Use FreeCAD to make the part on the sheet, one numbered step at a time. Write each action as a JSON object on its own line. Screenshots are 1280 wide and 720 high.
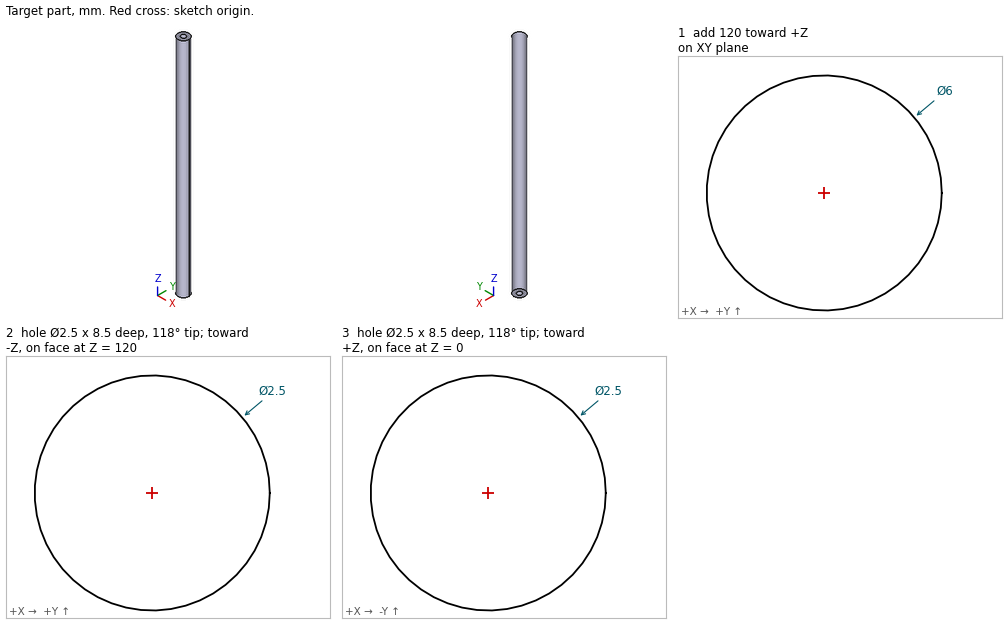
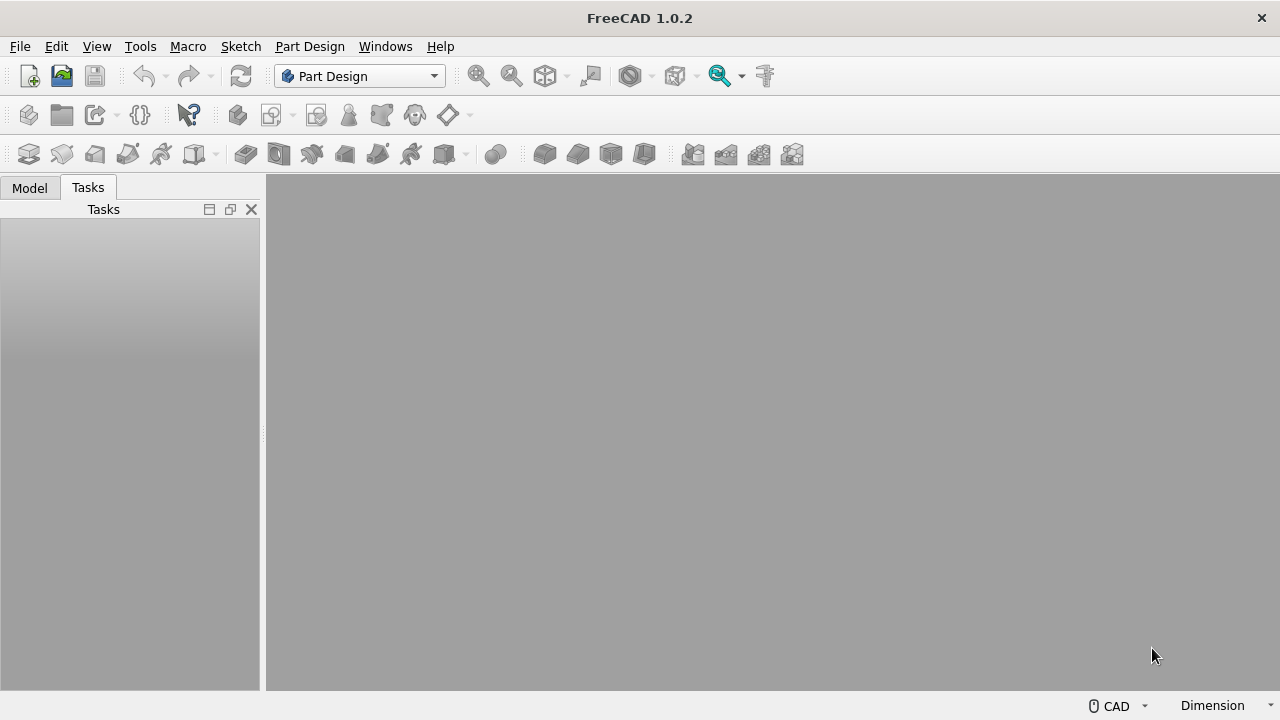
{"action": "left_click", "coordinate": [29, 76]}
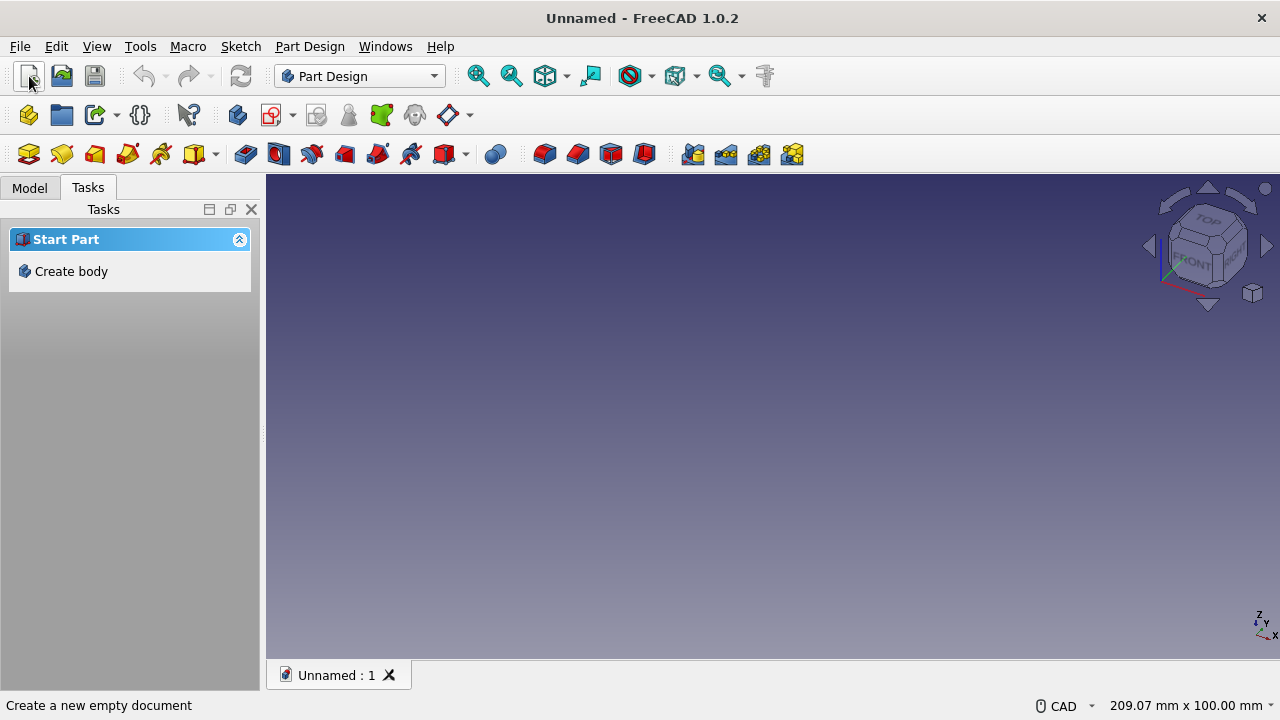
{"action": "left_click", "coordinate": [270, 116]}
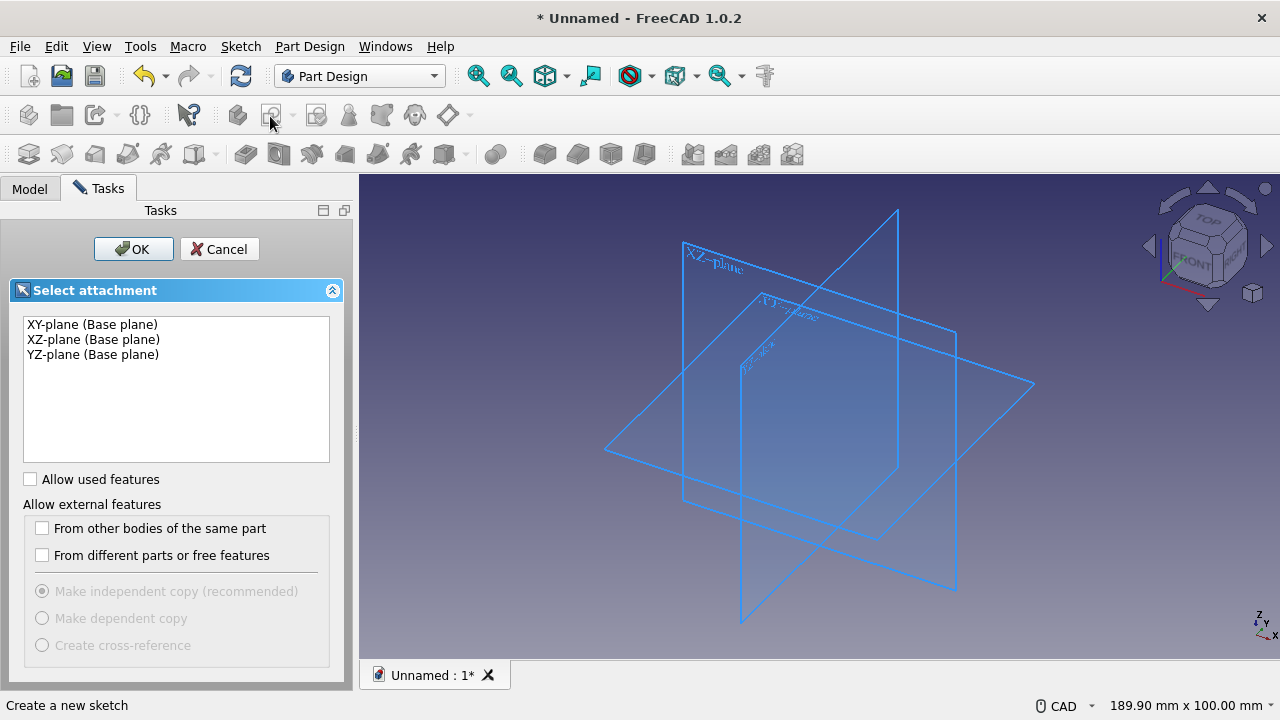
{"action": "left_click", "coordinate": [84, 324]}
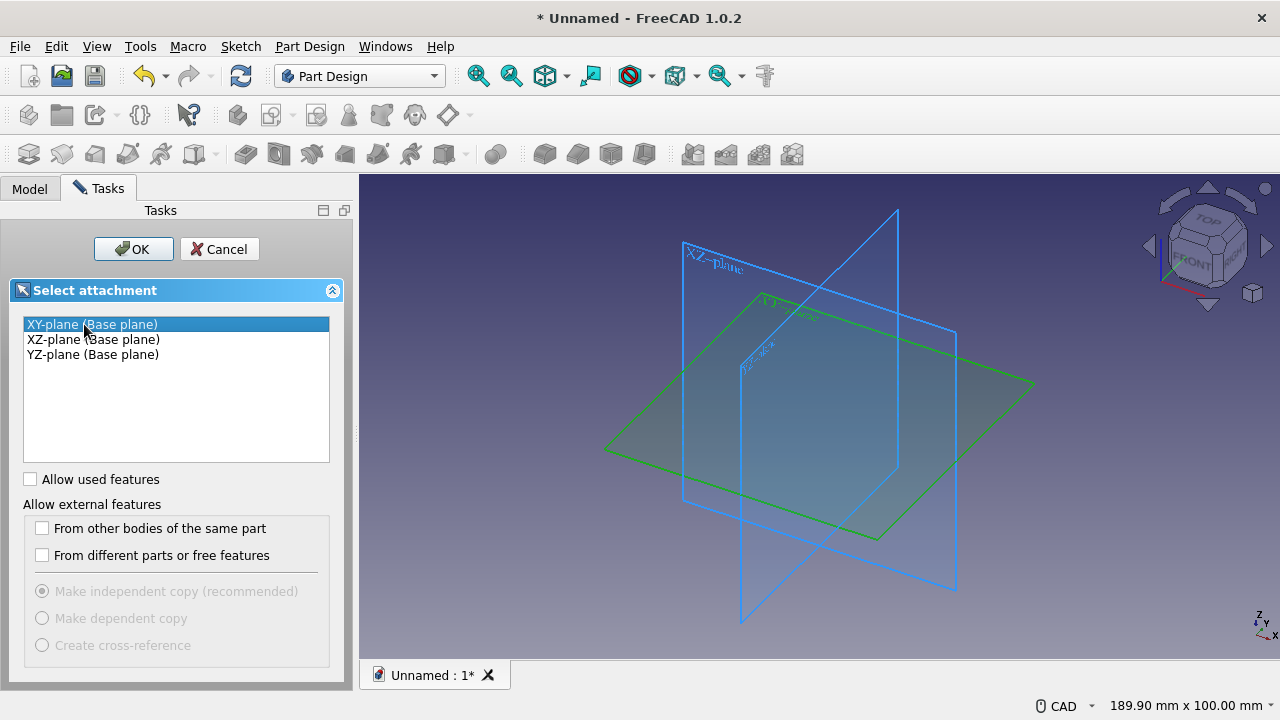
{"action": "left_click", "coordinate": [134, 249]}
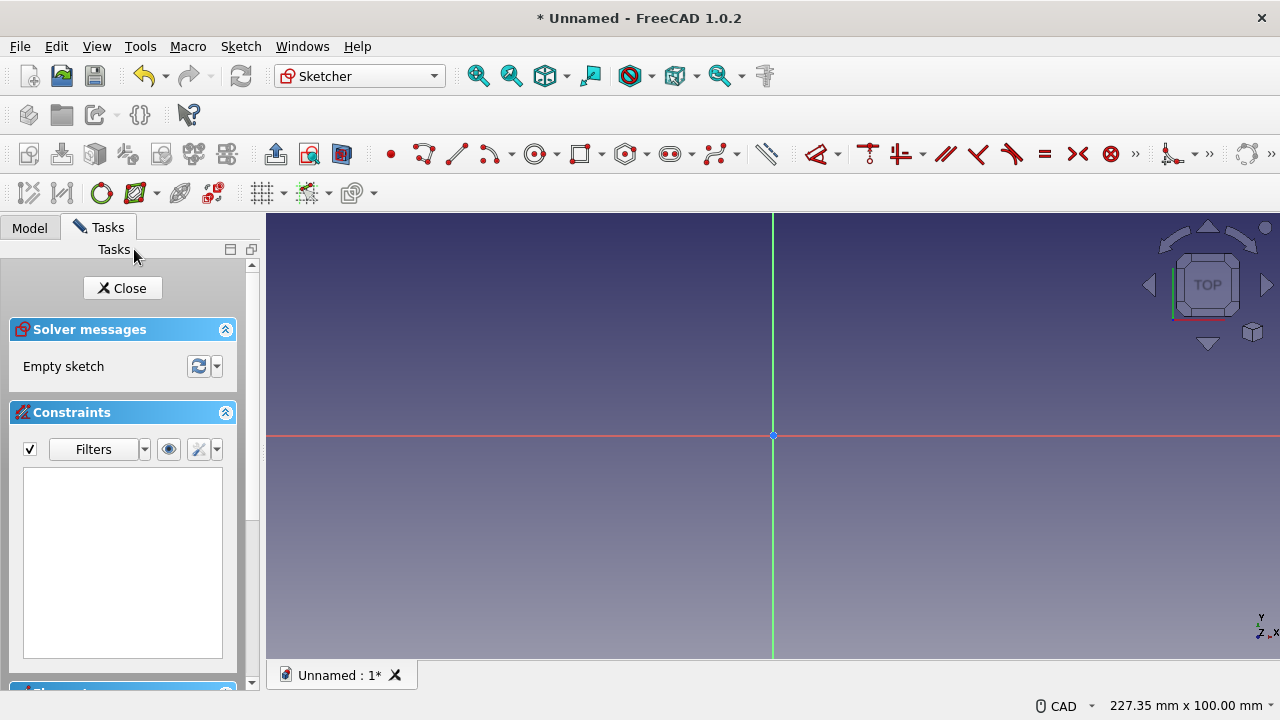
{"action": "scroll", "coordinate": [780, 436], "scroll_direction": "up", "scroll_amount": 12}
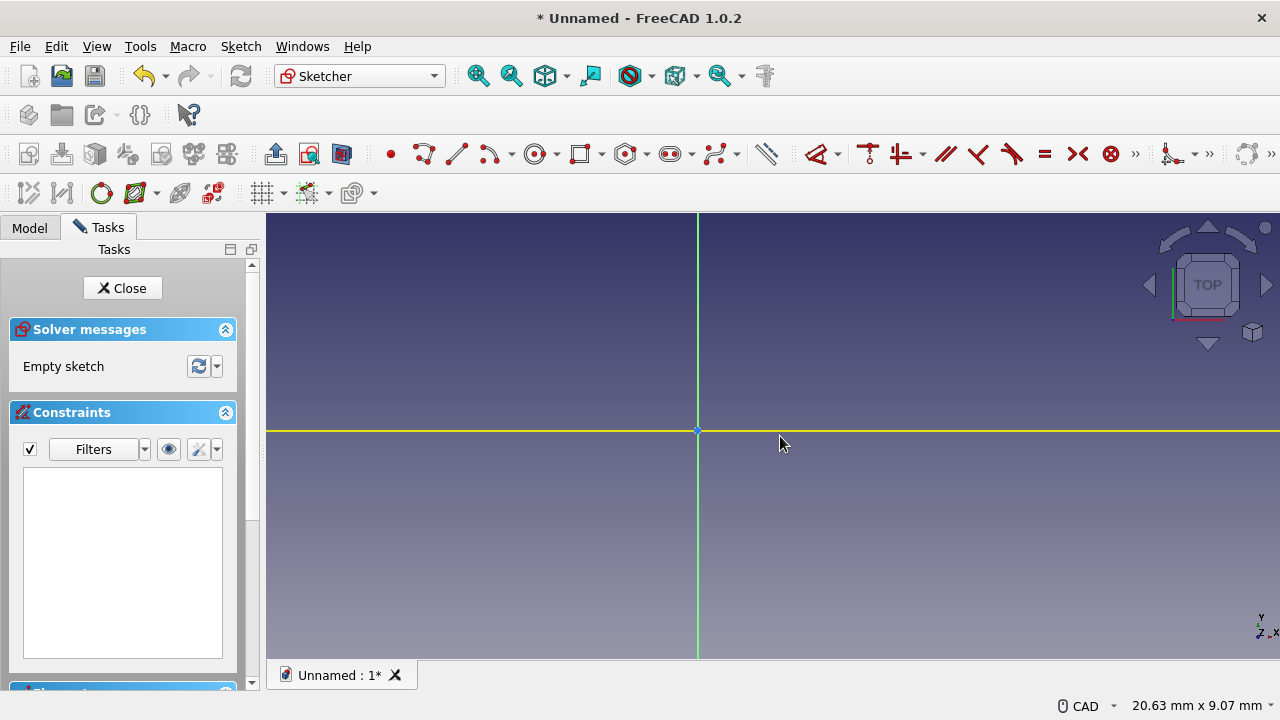
{"action": "left_click", "coordinate": [534, 154]}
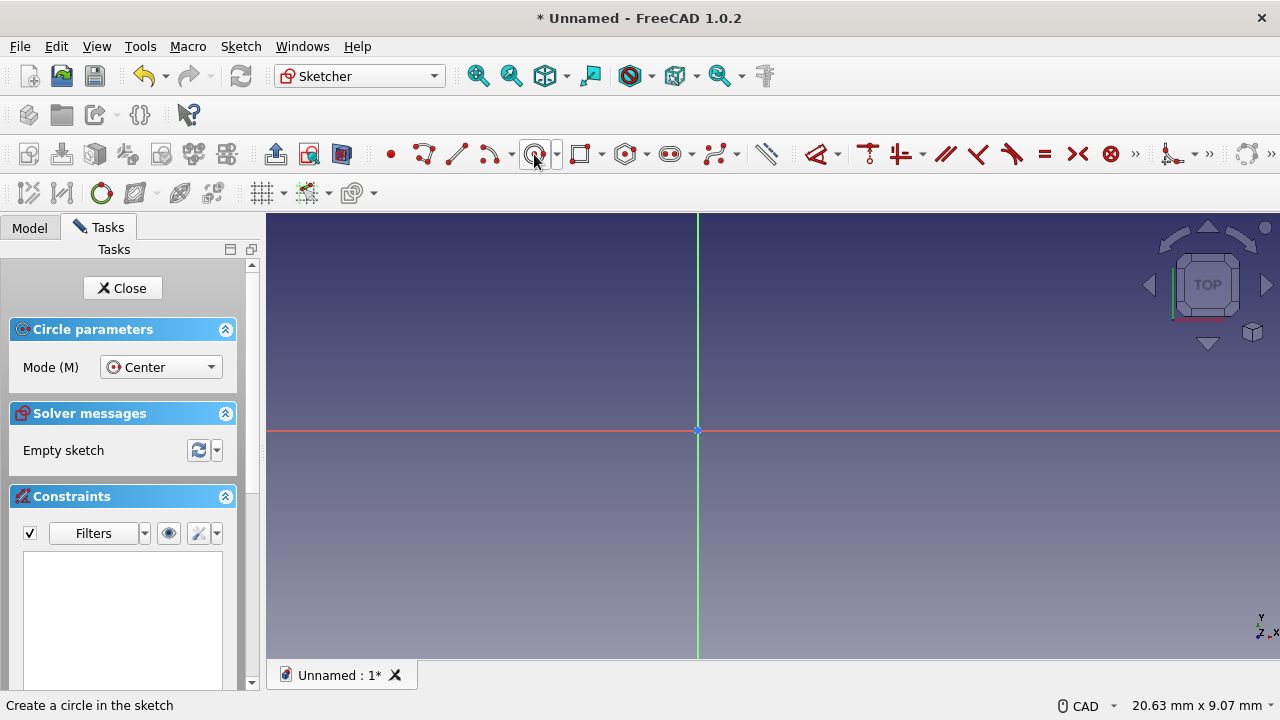
{"action": "left_click", "coordinate": [698, 431]}
{"action": "left_click", "coordinate": [802, 327]}
{"action": "key", "text": "Escape"}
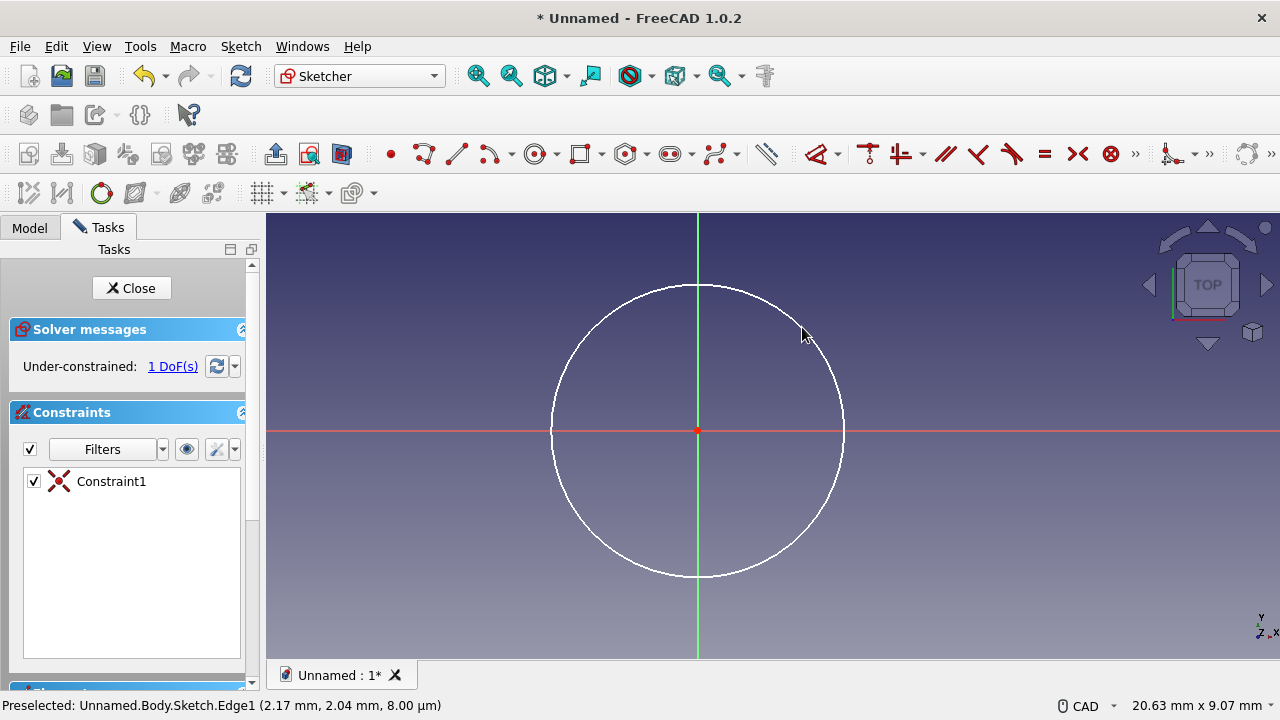
{"action": "left_click", "coordinate": [816, 154]}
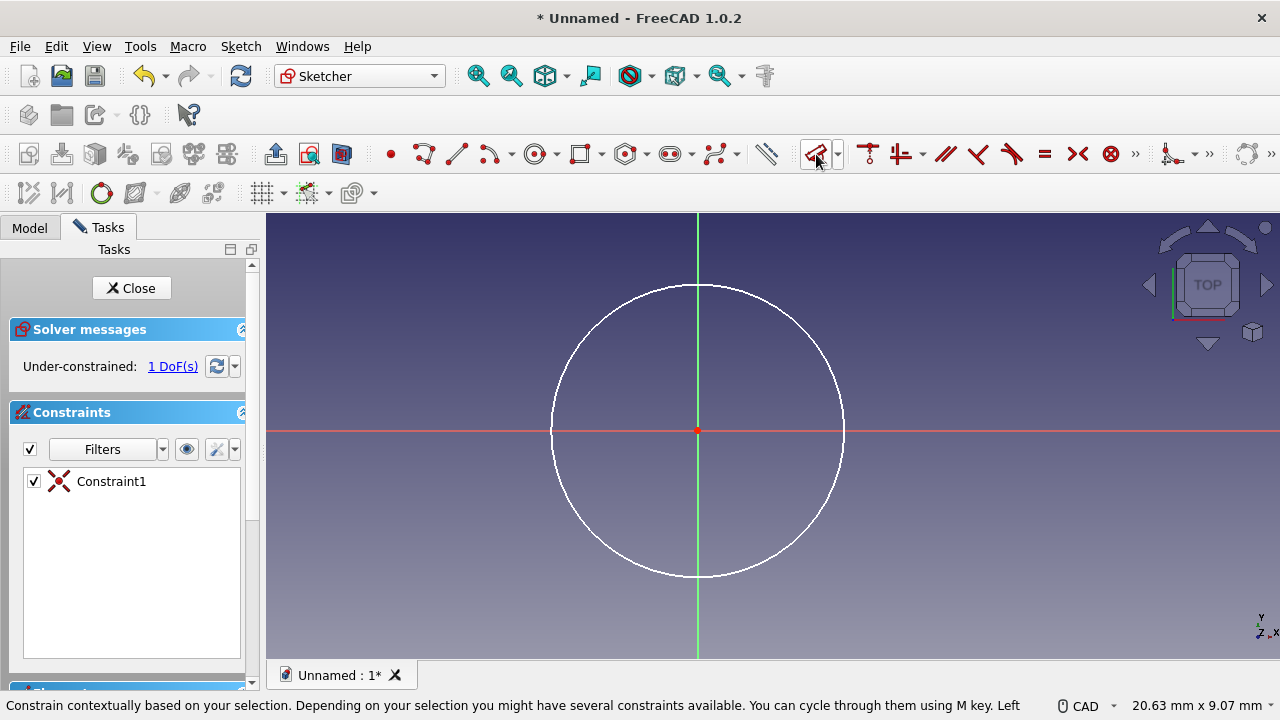
{"action": "left_click", "coordinate": [801, 327]}
{"action": "left_click", "coordinate": [824, 304]}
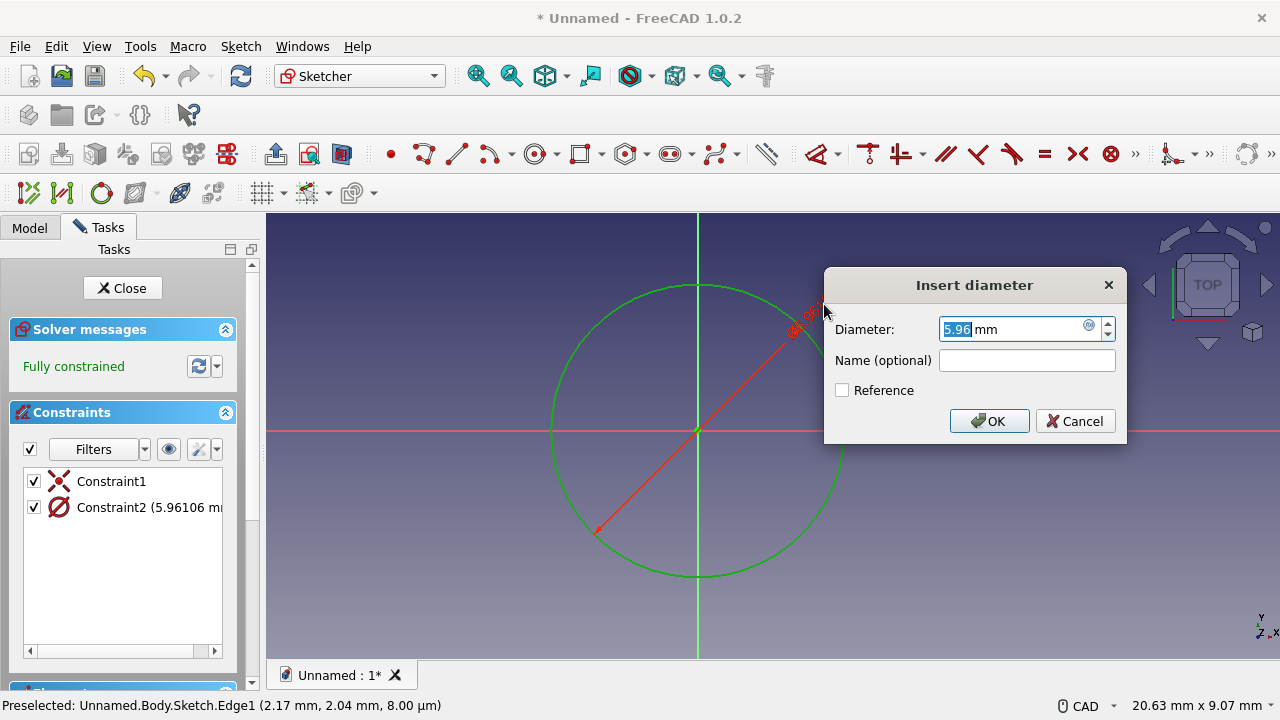
{"action": "type", "text": "6"}
{"action": "key", "text": "Return"}
{"action": "key", "text": "Escape"}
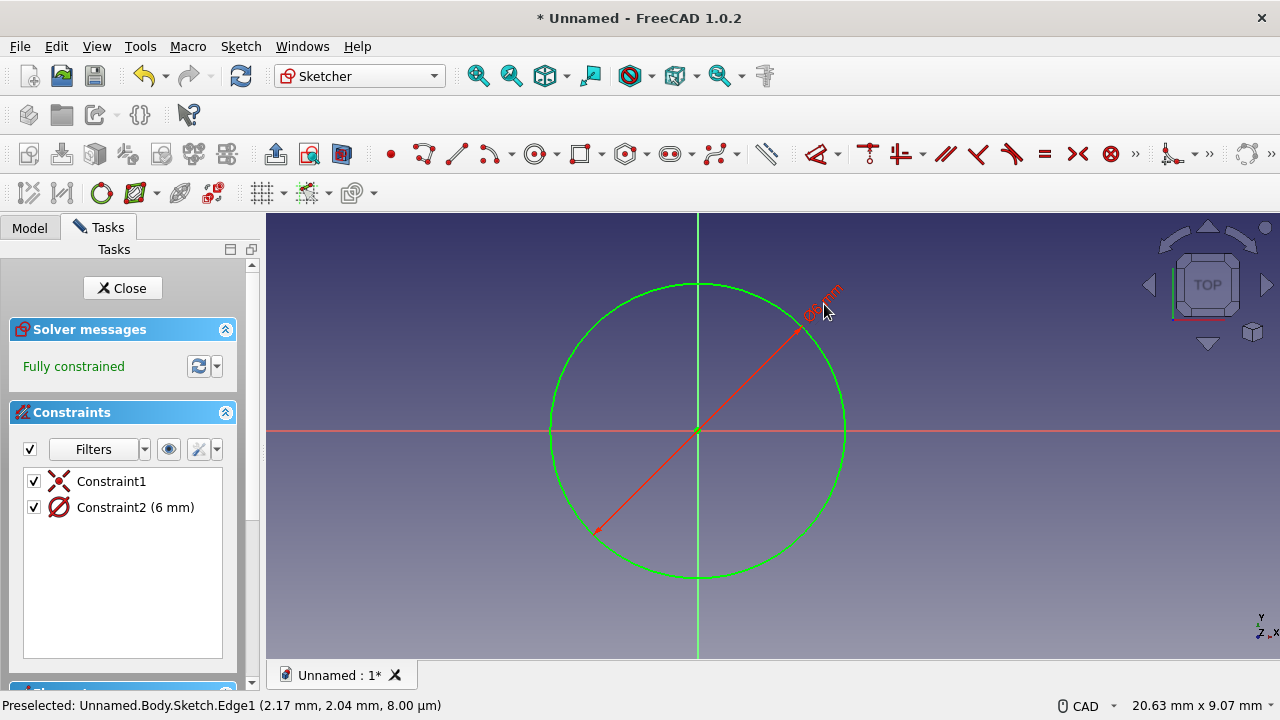
{"action": "left_click", "coordinate": [123, 288]}